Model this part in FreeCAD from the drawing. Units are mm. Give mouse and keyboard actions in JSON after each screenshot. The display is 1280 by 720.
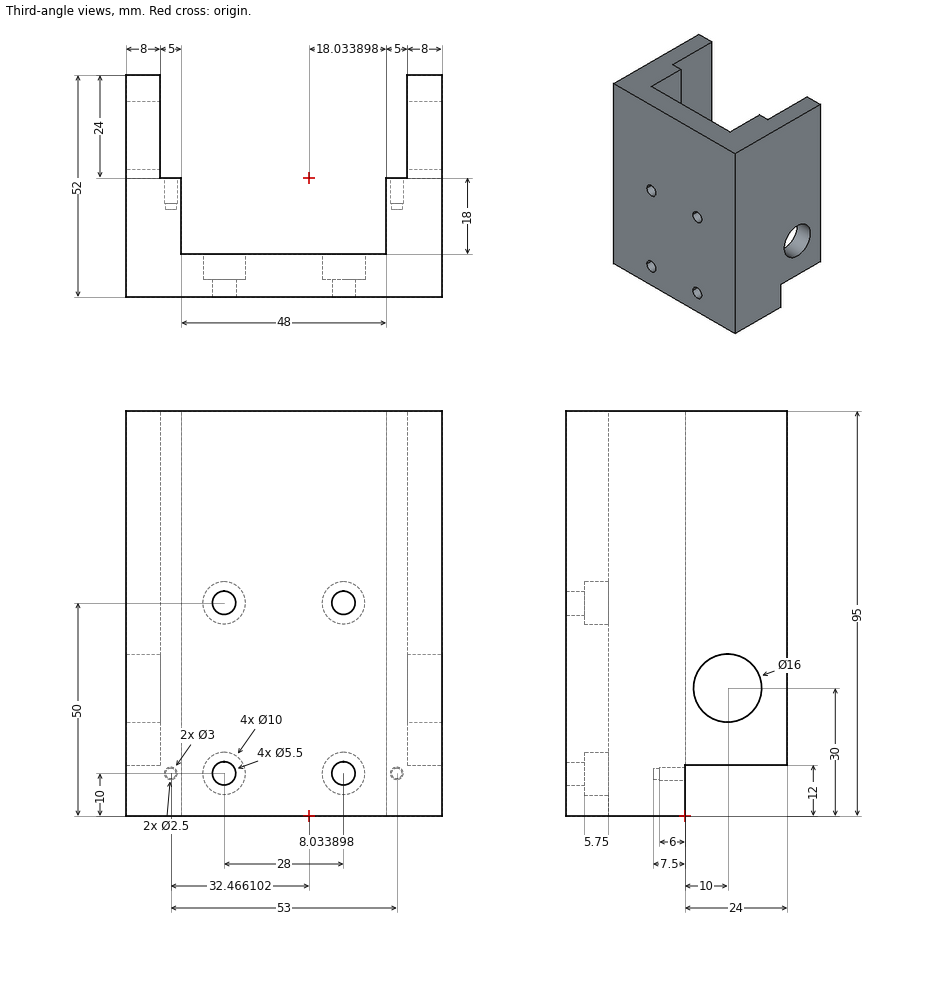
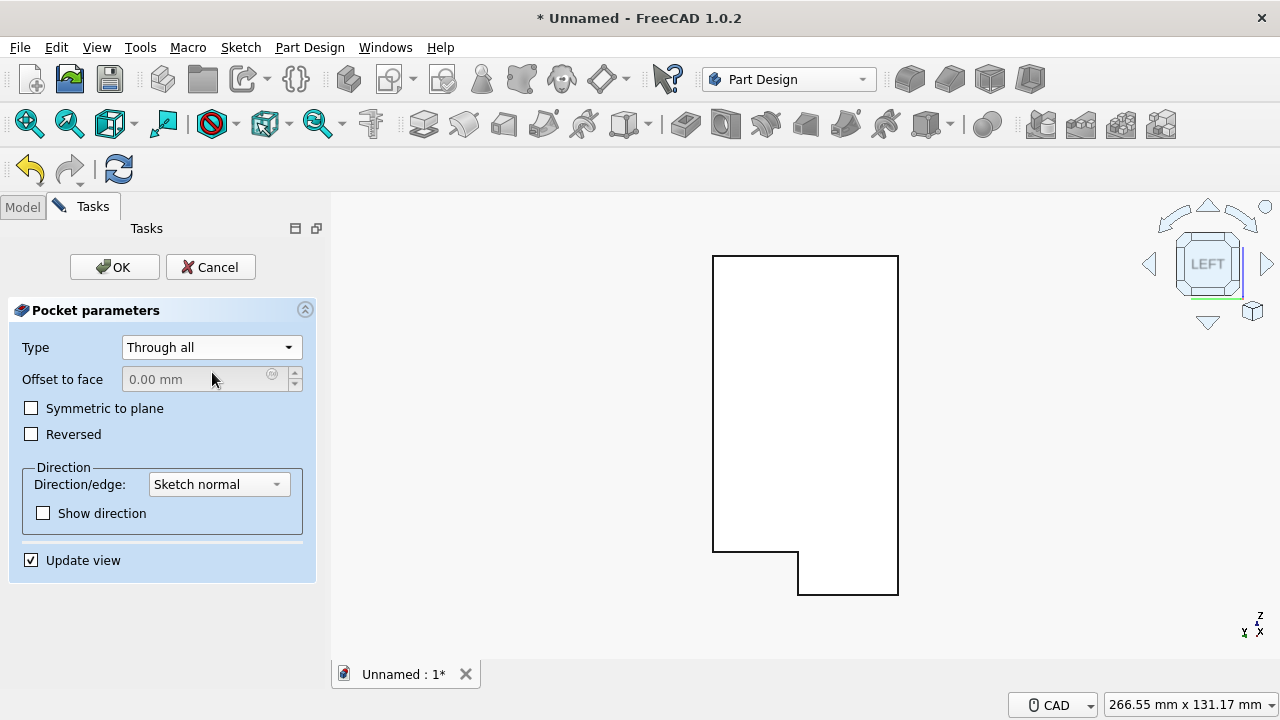
{"action": "left_click", "coordinate": [115, 267]}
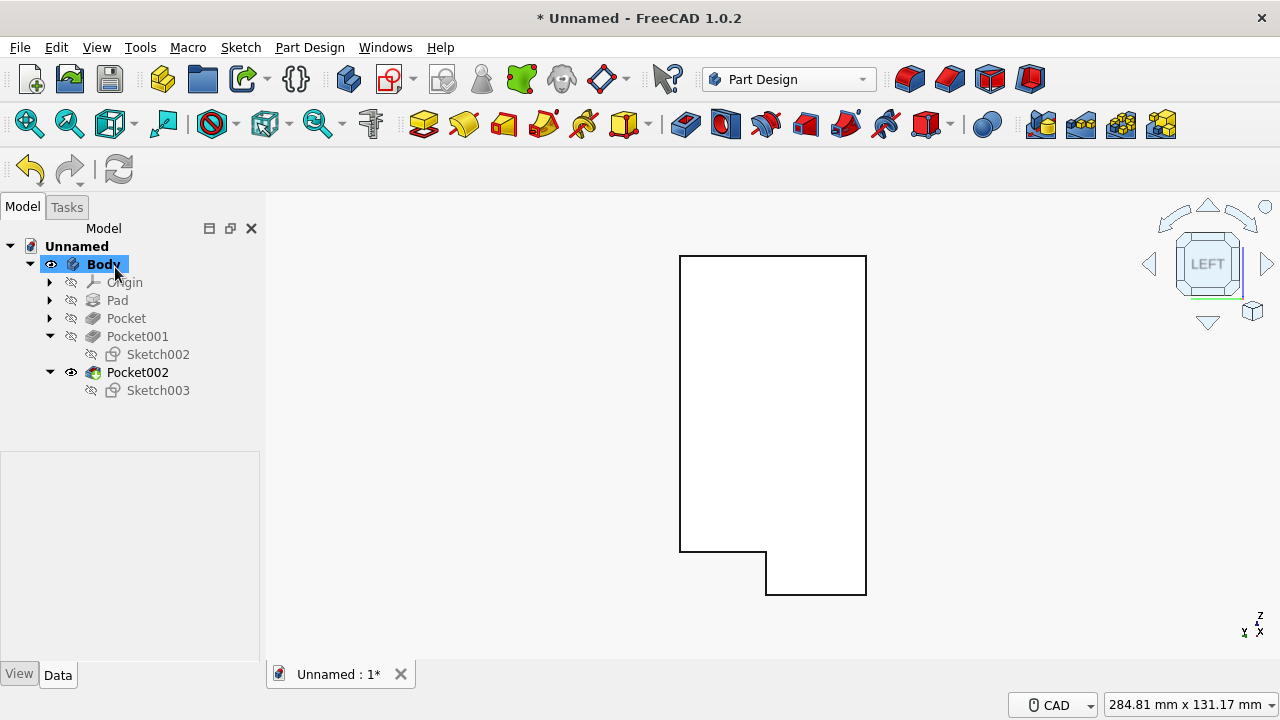
{"action": "left_click", "coordinate": [390, 80]}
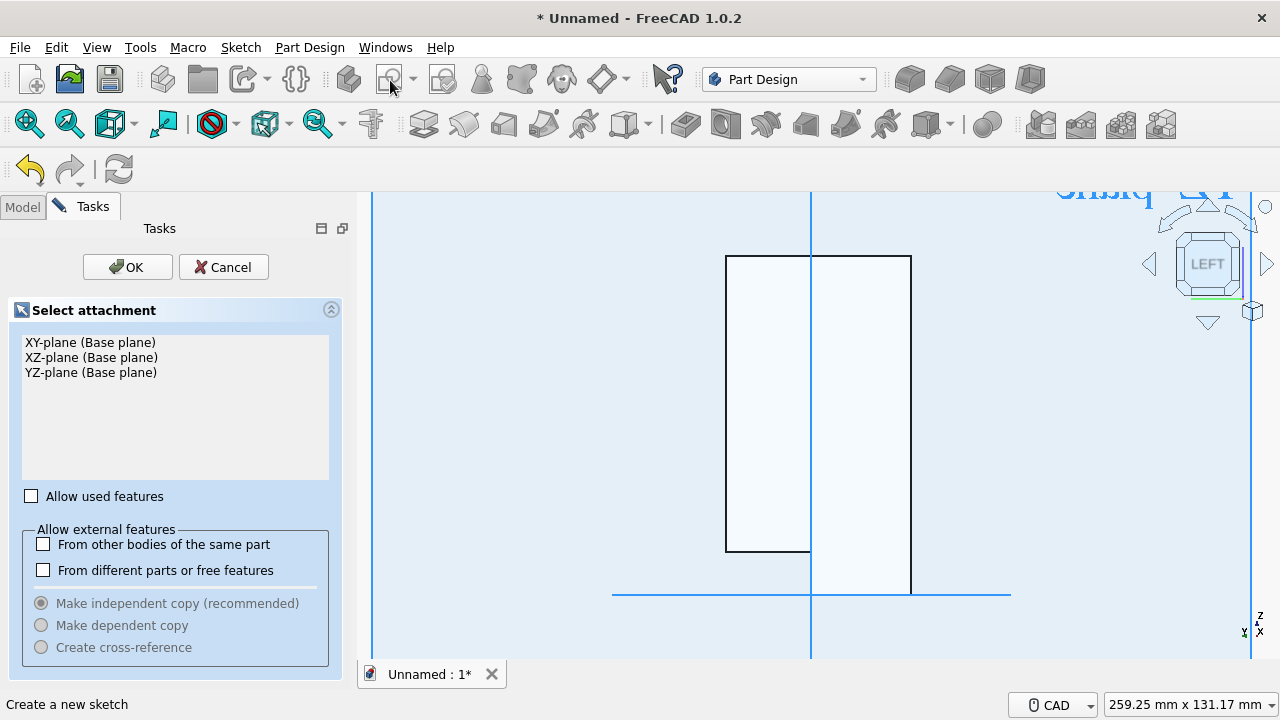
{"action": "left_click", "coordinate": [82, 358]}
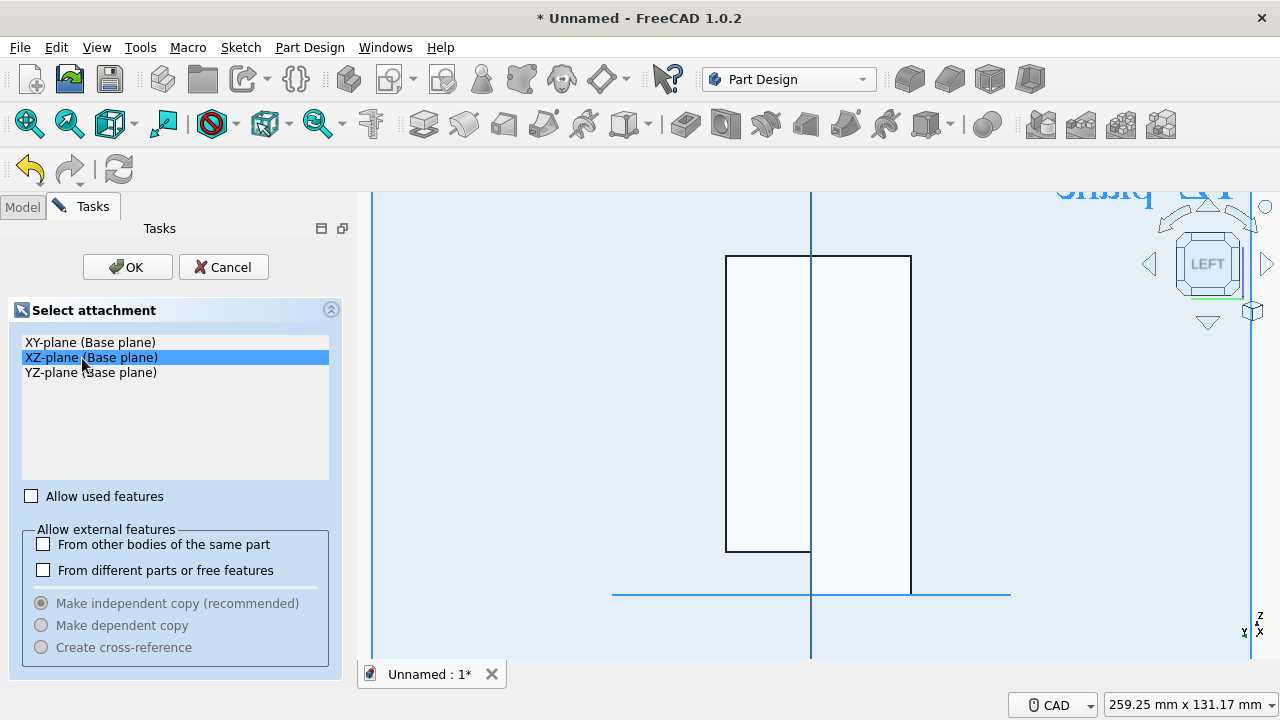
{"action": "left_click", "coordinate": [128, 267]}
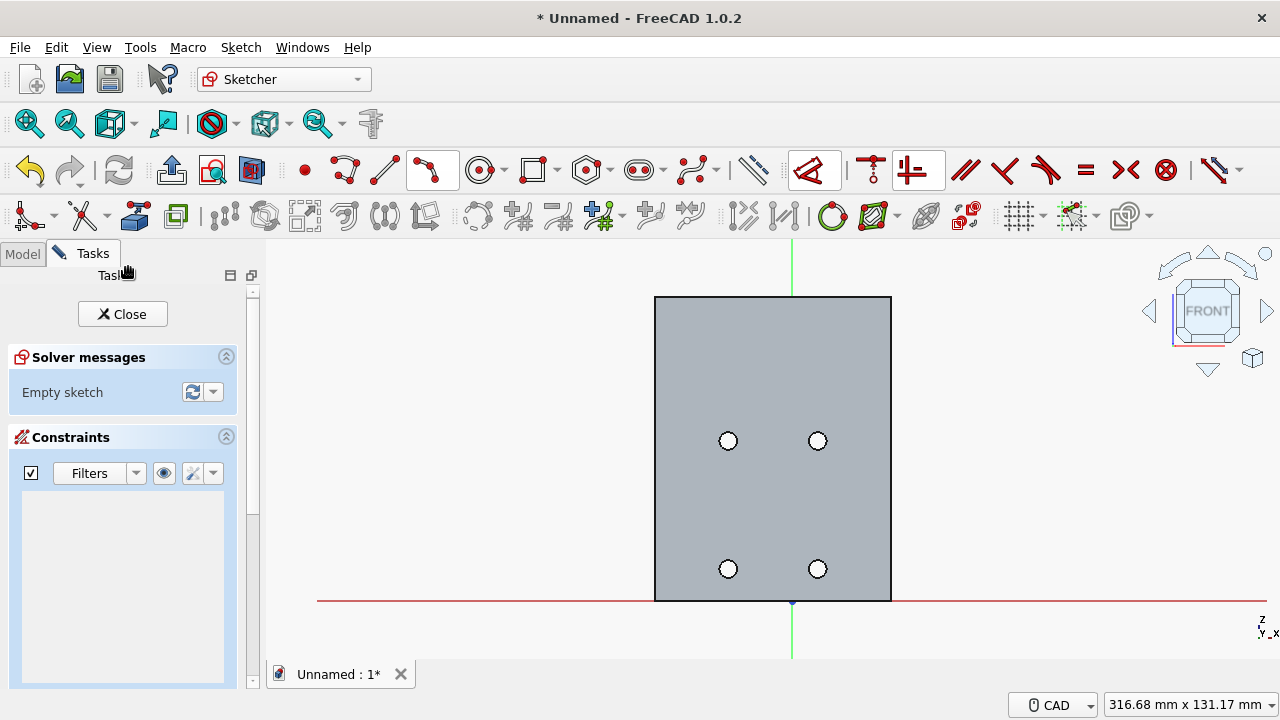
{"action": "key", "text": "q s"}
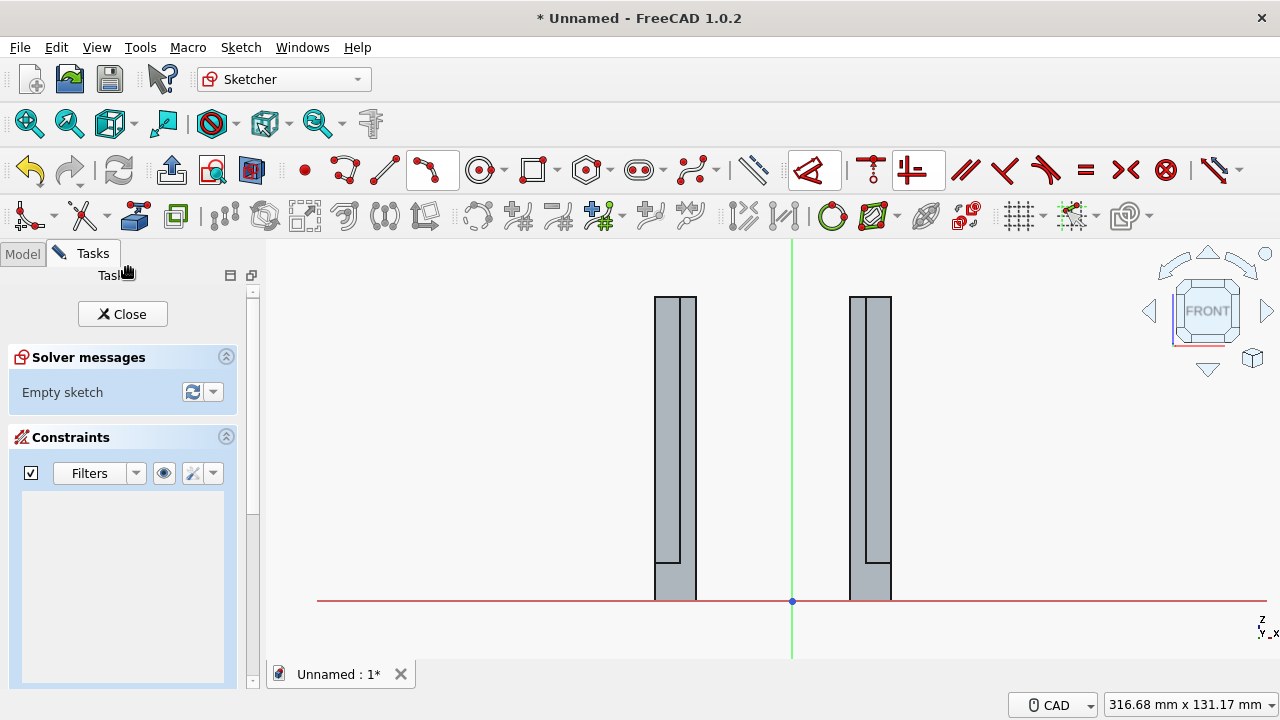
{"action": "scroll", "coordinate": [803, 631], "scroll_direction": "up", "scroll_amount": 6}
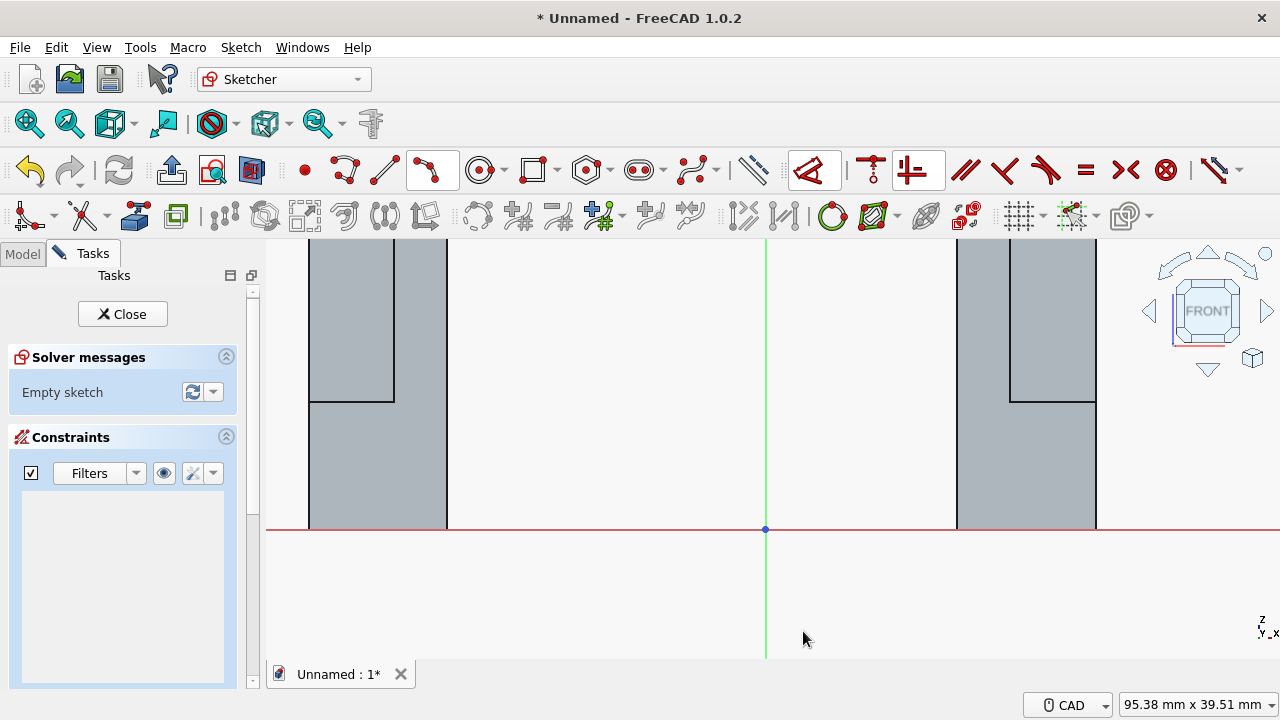
{"action": "key", "text": "g c"}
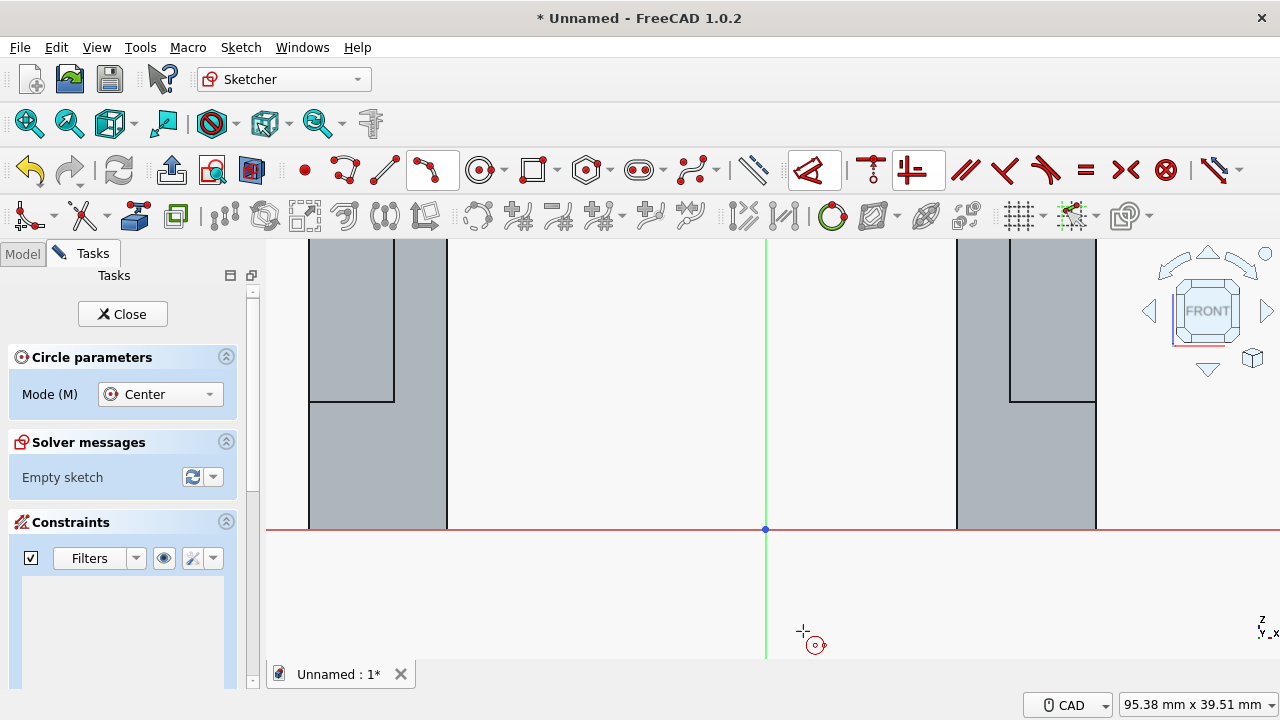
{"action": "scroll", "coordinate": [420, 423], "scroll_direction": "up", "scroll_amount": 3}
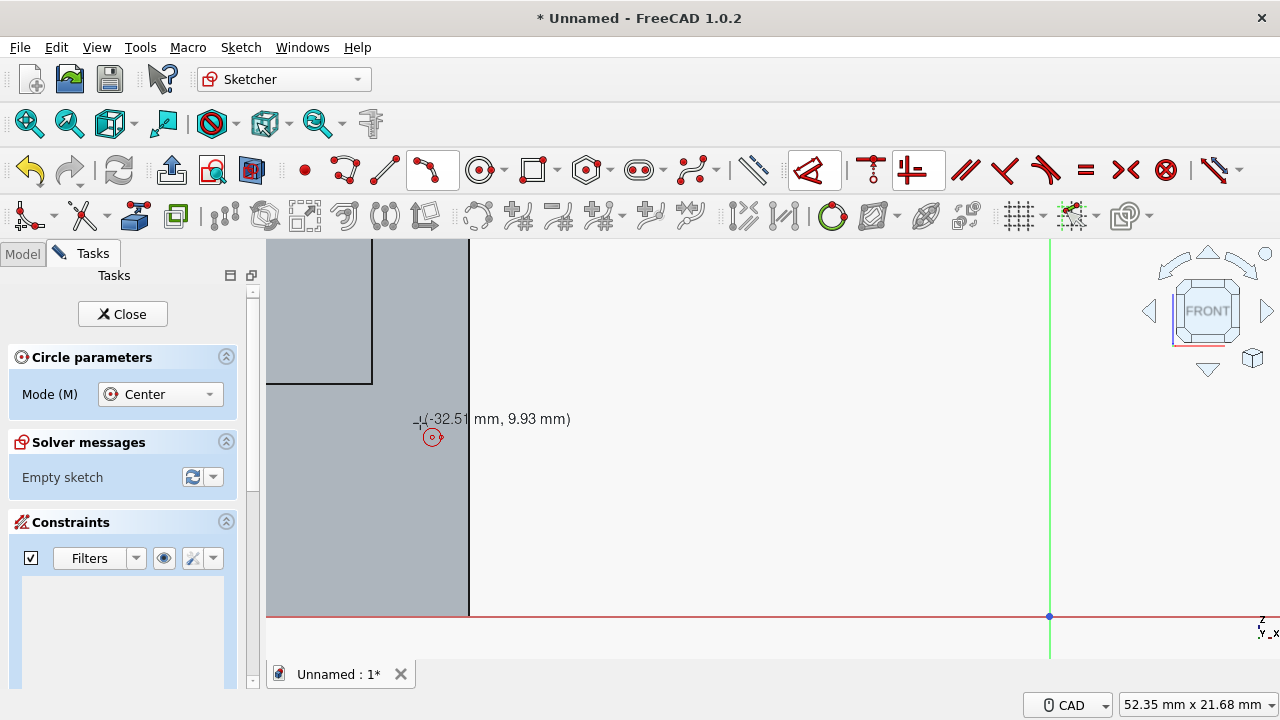
{"action": "left_click", "coordinate": [421, 423]}
{"action": "left_click", "coordinate": [438, 406]}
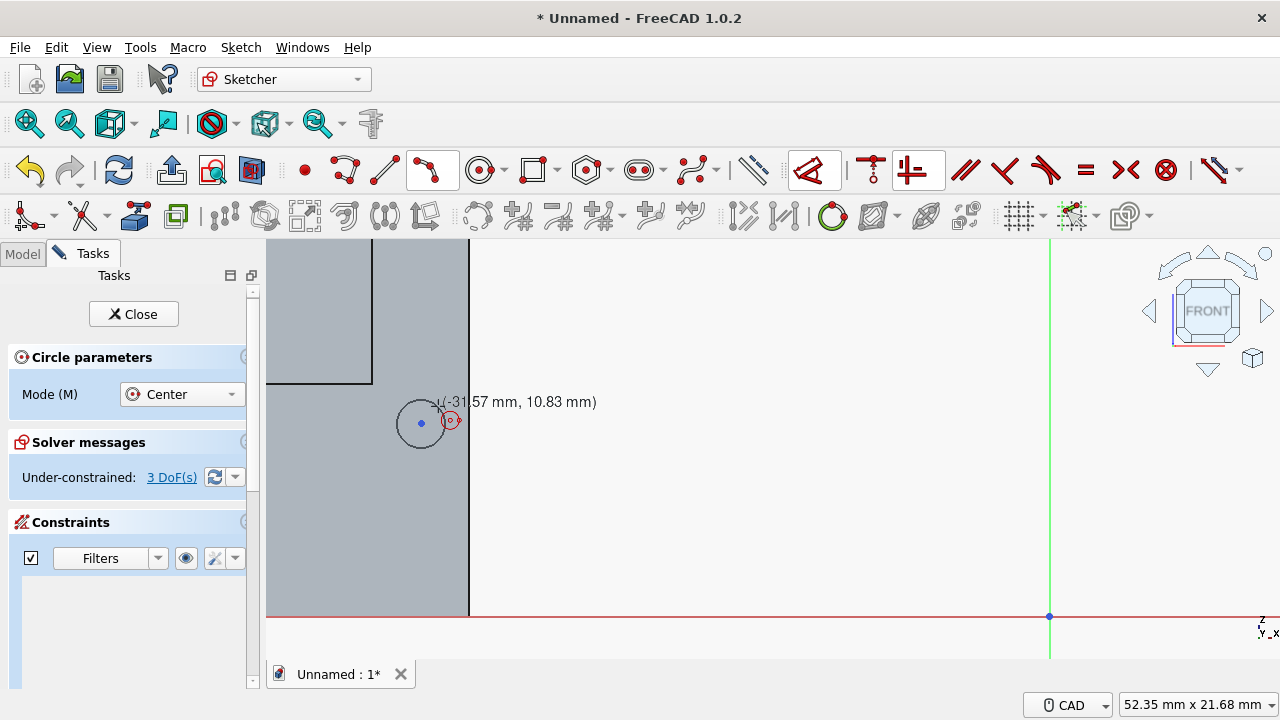
{"action": "scroll", "coordinate": [425, 377], "scroll_direction": "down", "scroll_amount": 3}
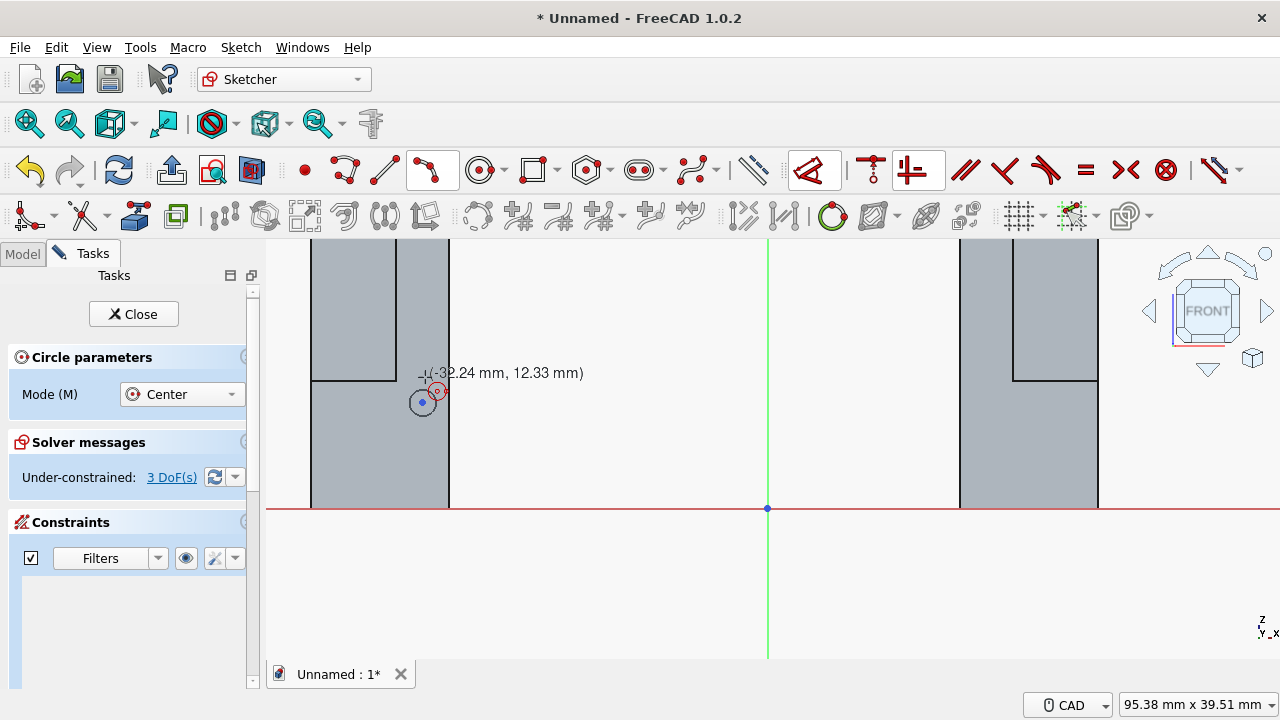
{"action": "scroll", "coordinate": [986, 402], "scroll_direction": "up", "scroll_amount": 3}